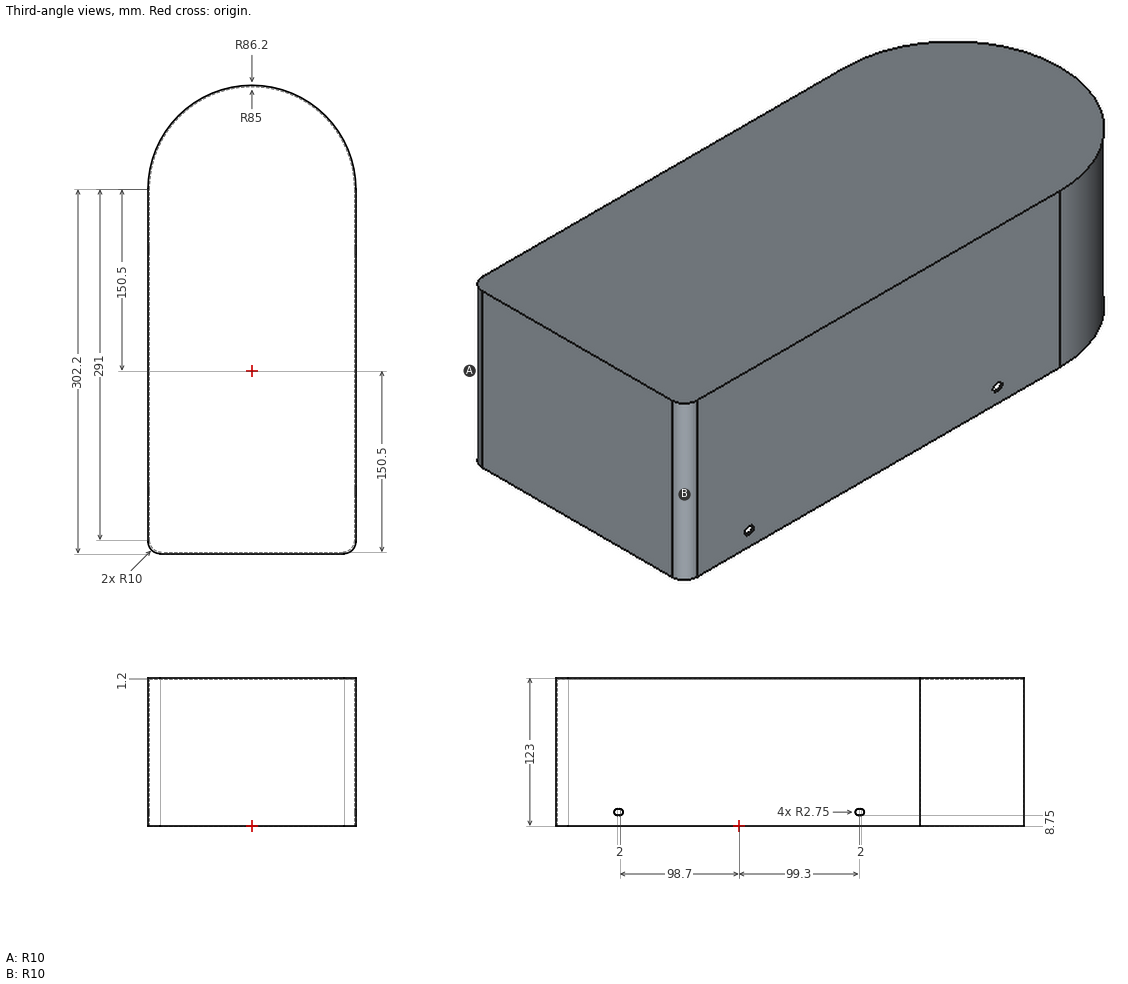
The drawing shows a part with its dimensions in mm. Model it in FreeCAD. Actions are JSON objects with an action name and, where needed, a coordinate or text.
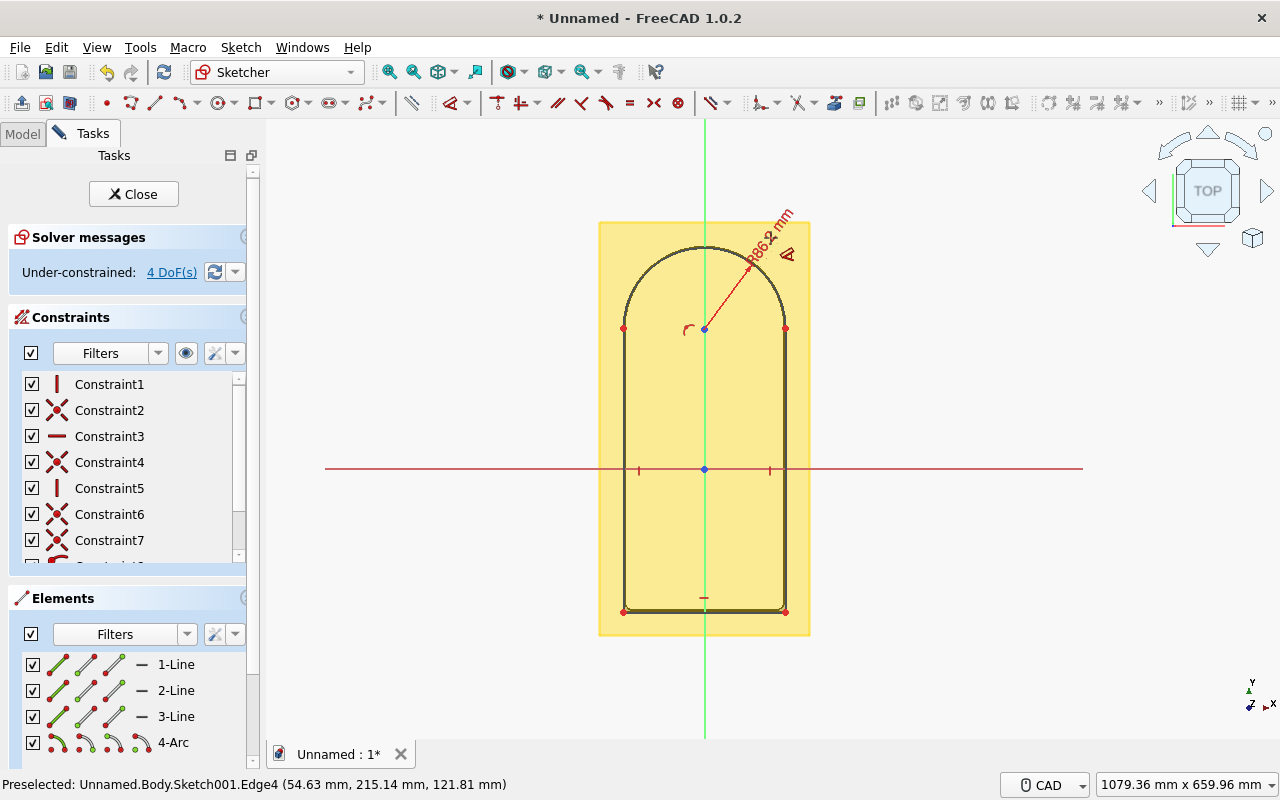
{"action": "left_click", "coordinate": [624, 414]}
{"action": "left_click", "coordinate": [590, 406]}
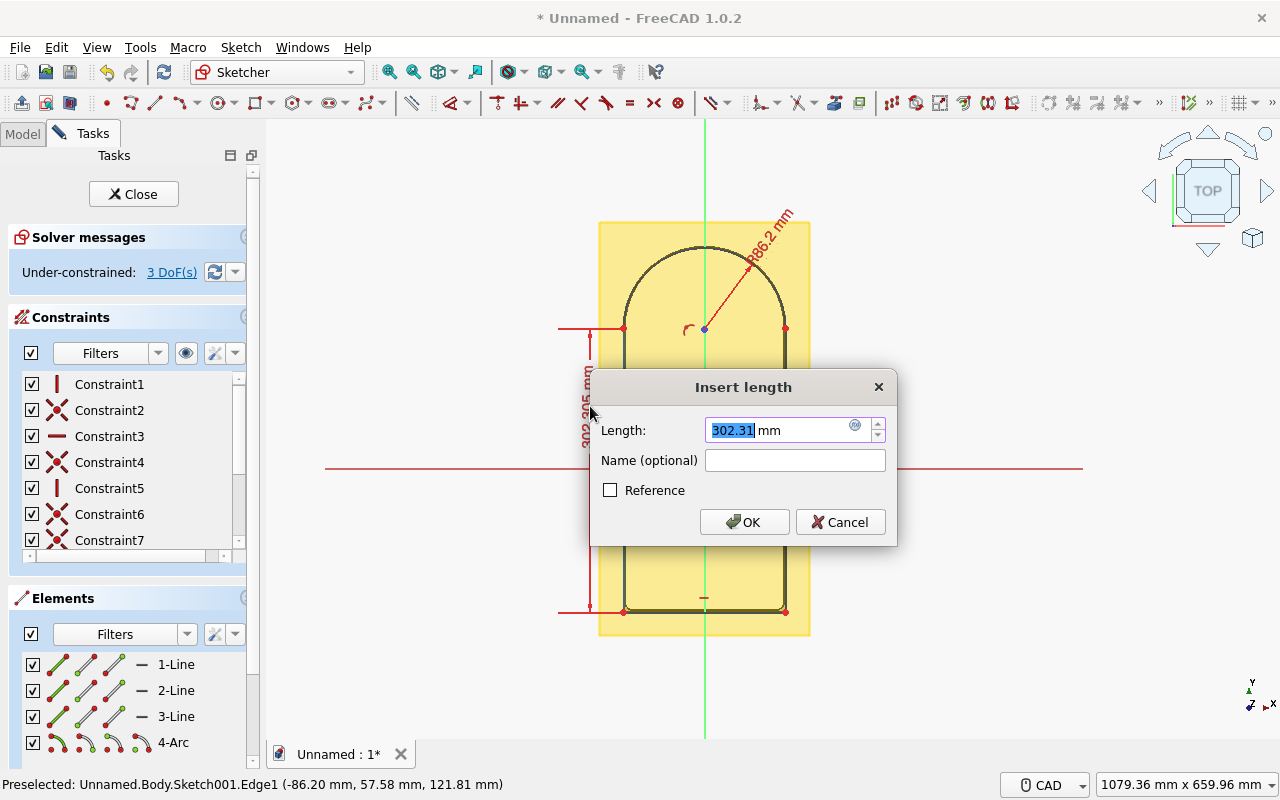
{"action": "type", "text": "302.2"}
{"action": "key", "text": "Return"}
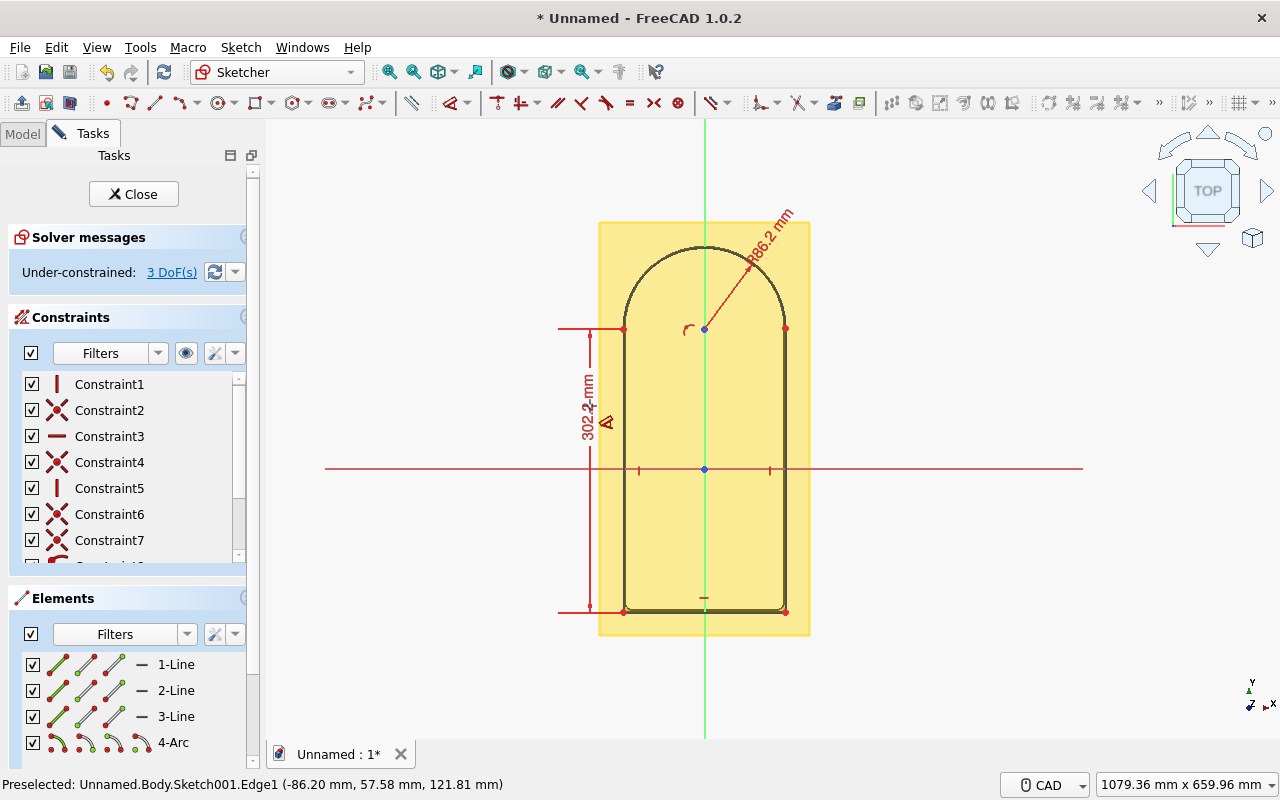
{"action": "left_click", "coordinate": [786, 528]}
{"action": "left_click", "coordinate": [820, 406]}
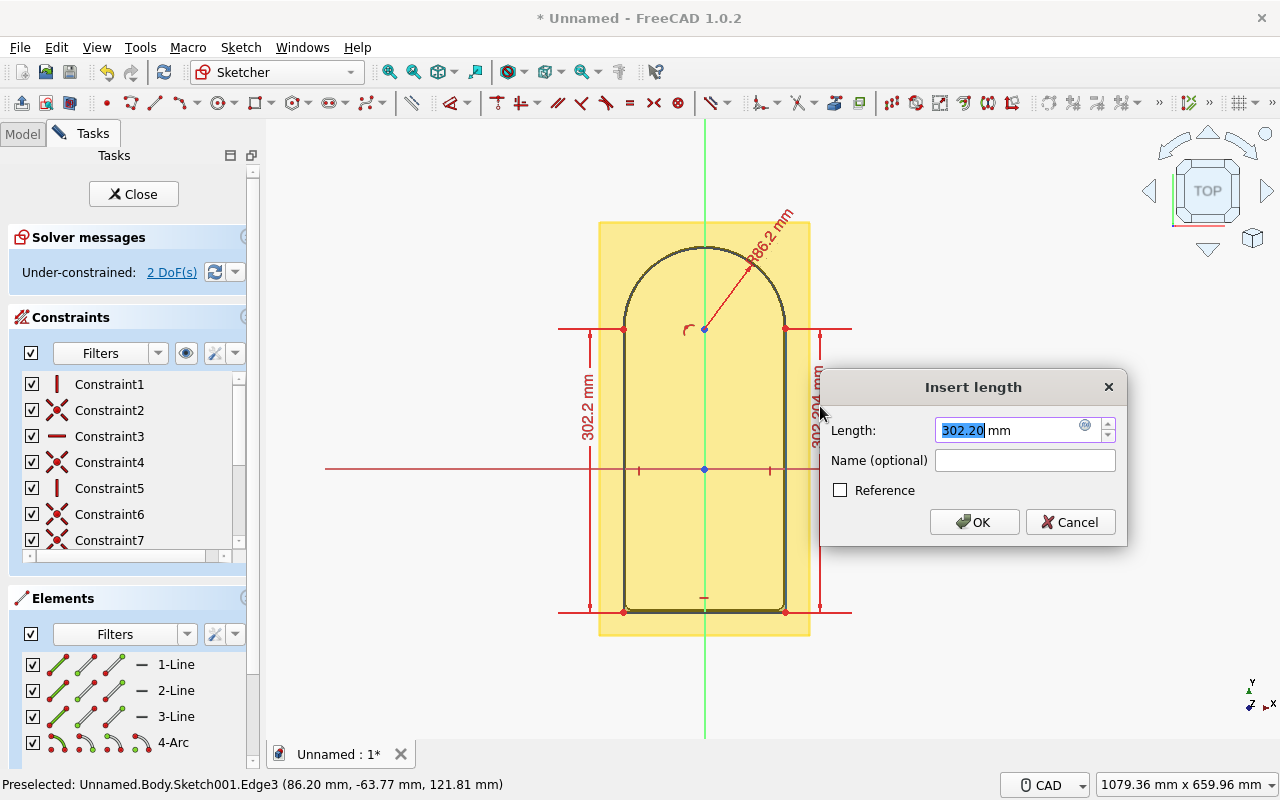
{"action": "type", "text": "302.2"}
{"action": "key", "text": "Return"}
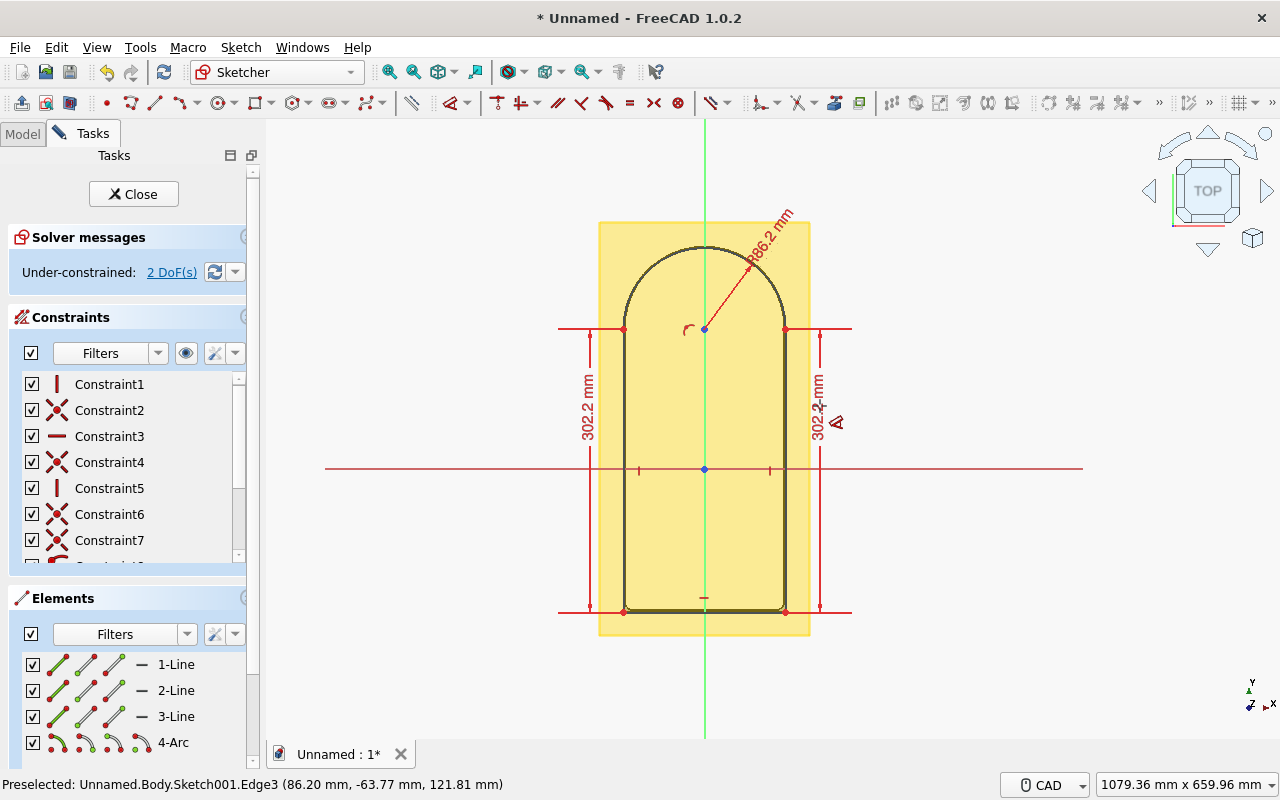
{"action": "left_click", "coordinate": [624, 329]}
{"action": "left_click", "coordinate": [590, 367]}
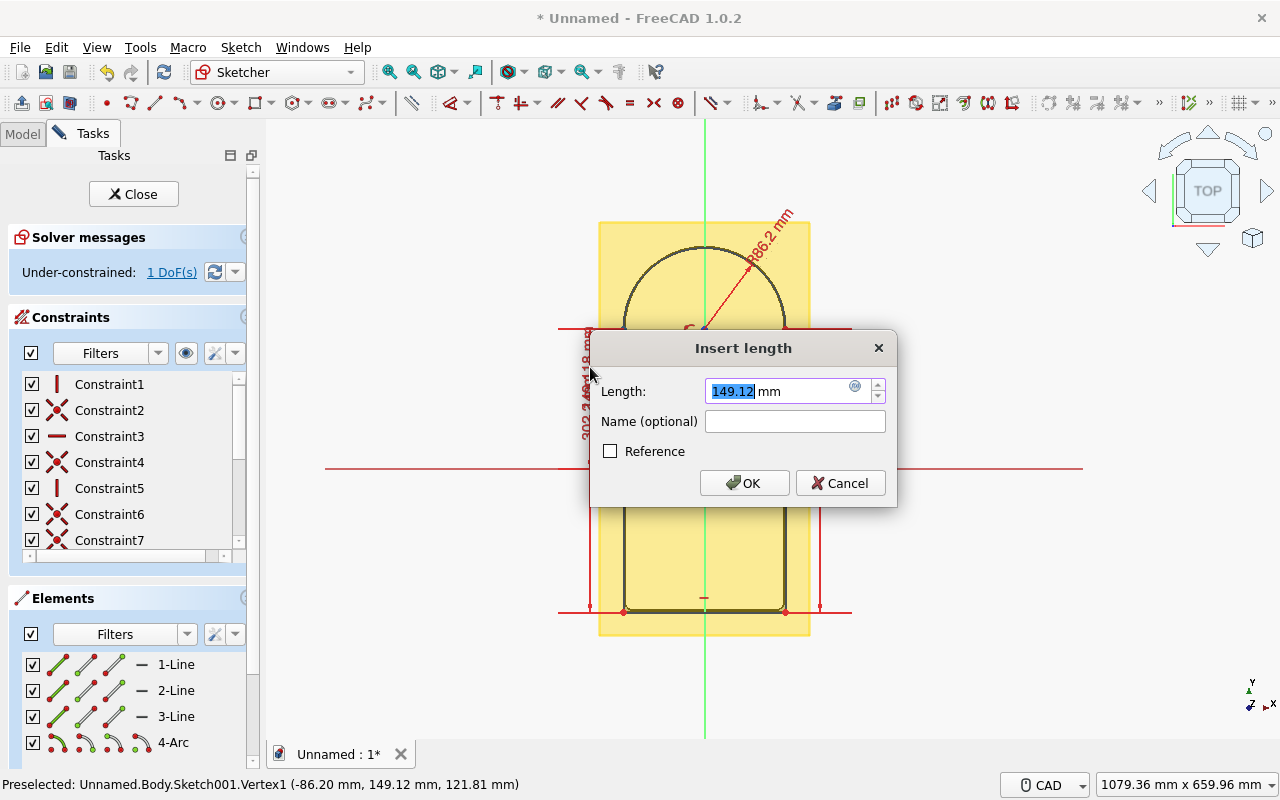
{"action": "type", "text": "150.5"}
{"action": "key", "text": "Return"}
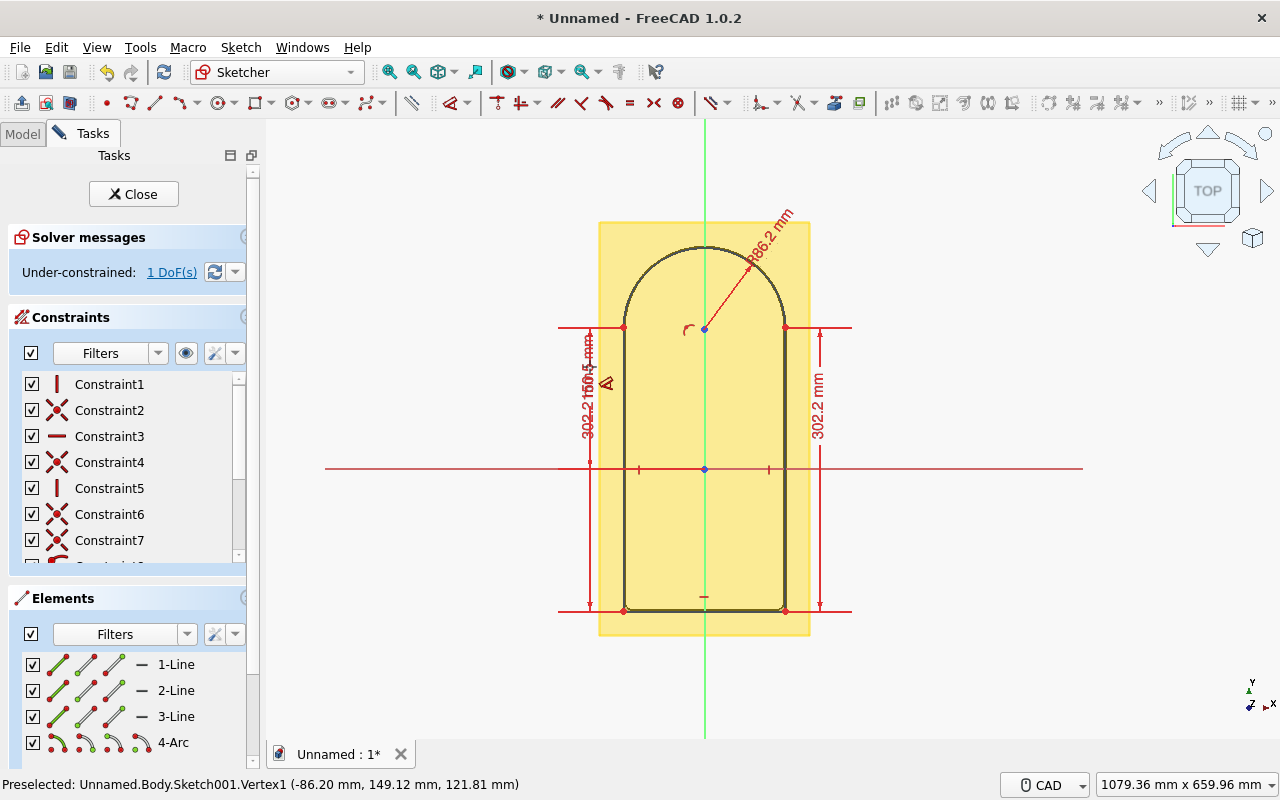
{"action": "left_click", "coordinate": [705, 329]}
{"action": "left_click", "coordinate": [739, 399]}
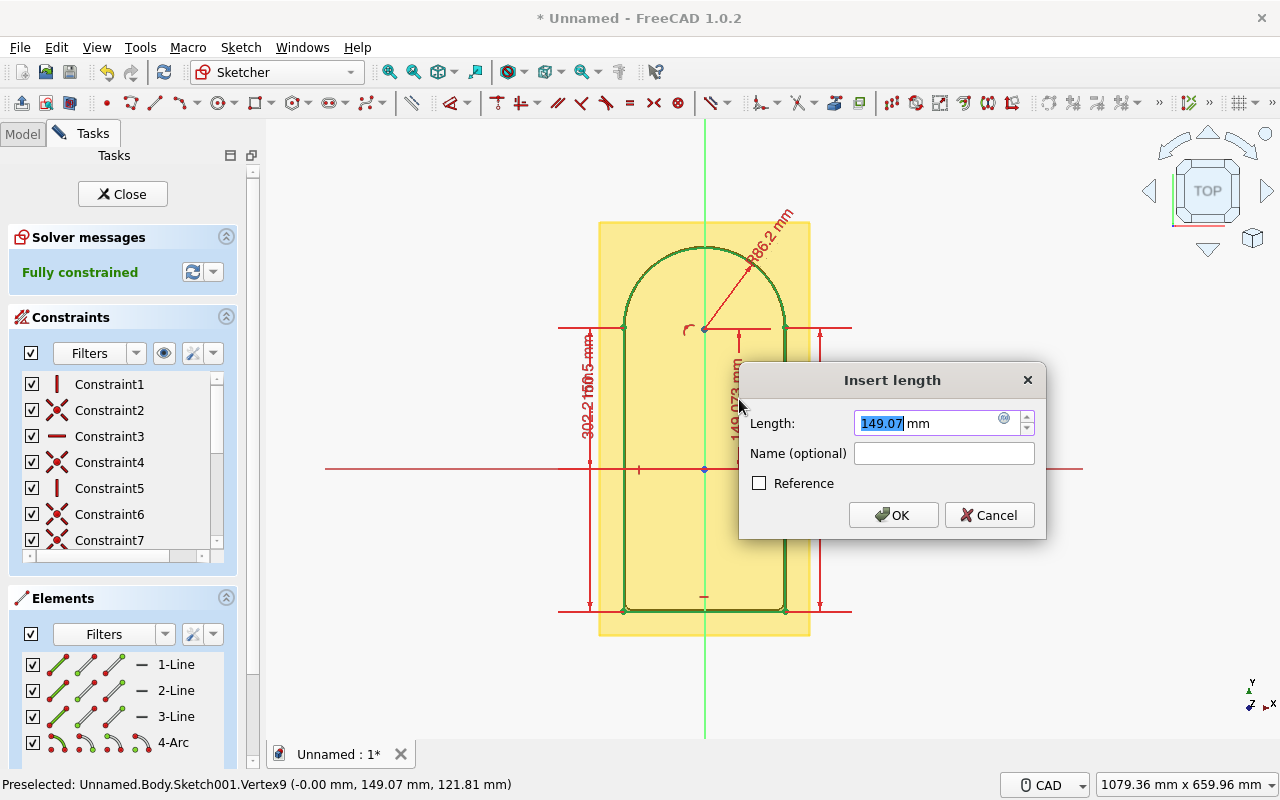
{"action": "type", "text": "150.5"}
{"action": "key", "text": "Return"}
{"action": "key", "text": "Escape"}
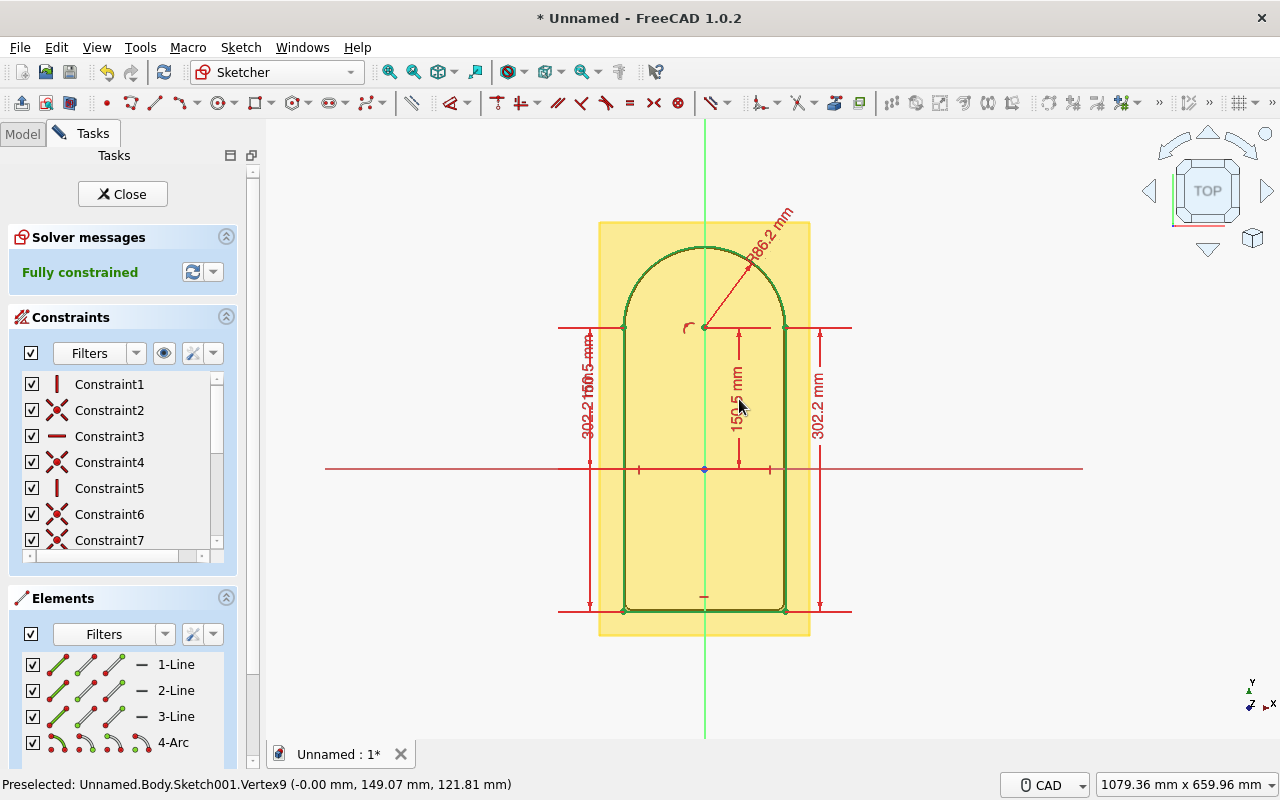
{"action": "left_click", "coordinate": [123, 194]}